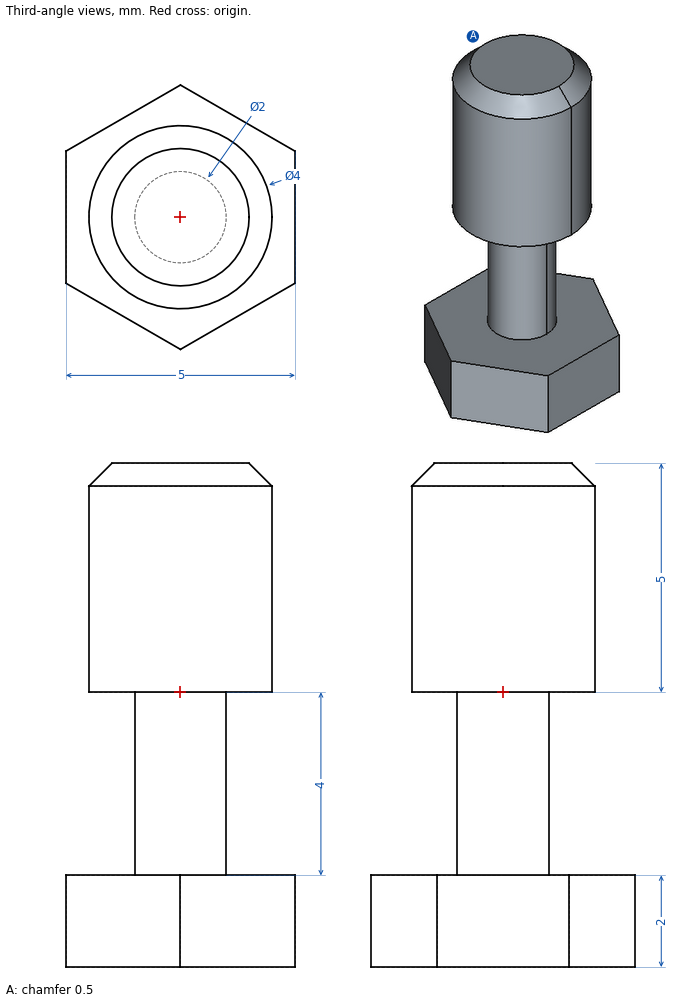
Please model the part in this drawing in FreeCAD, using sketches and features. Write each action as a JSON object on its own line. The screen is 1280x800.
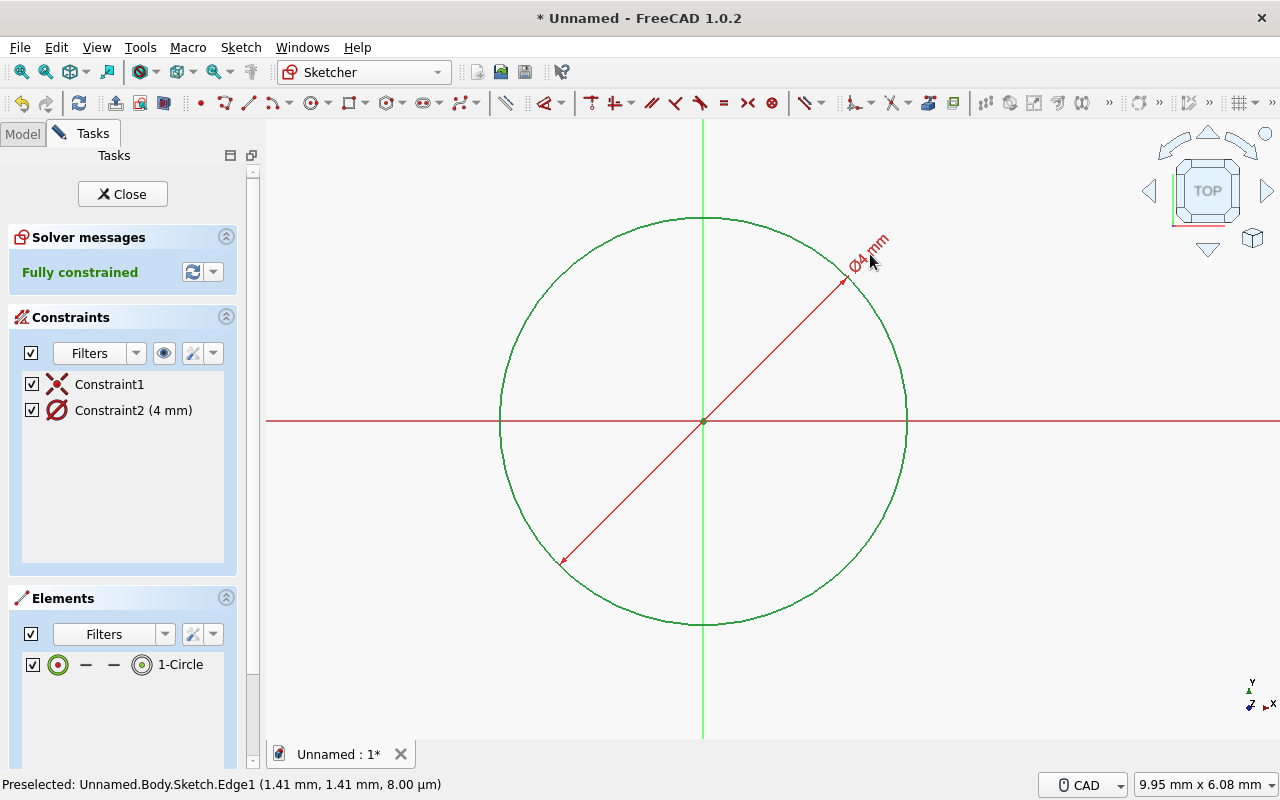
{"action": "left_click", "coordinate": [123, 194]}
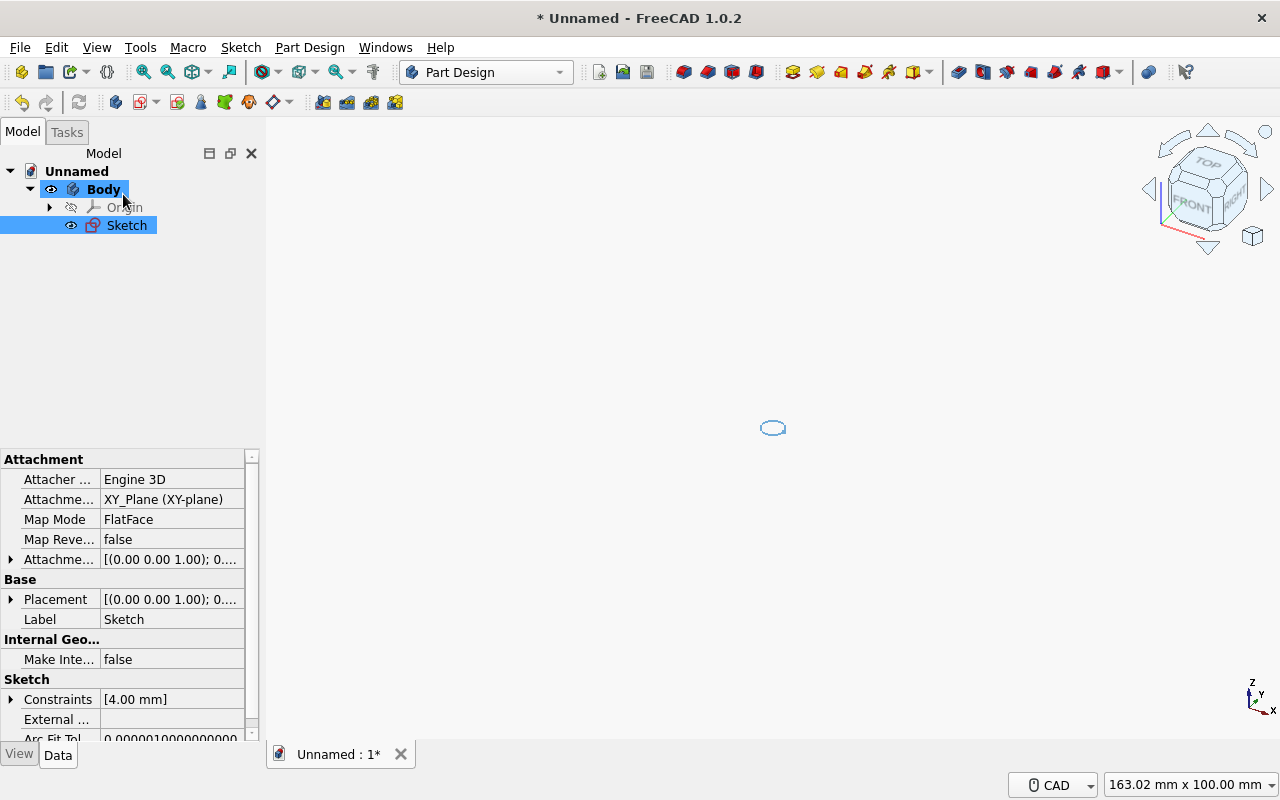
{"action": "left_click", "coordinate": [794, 72]}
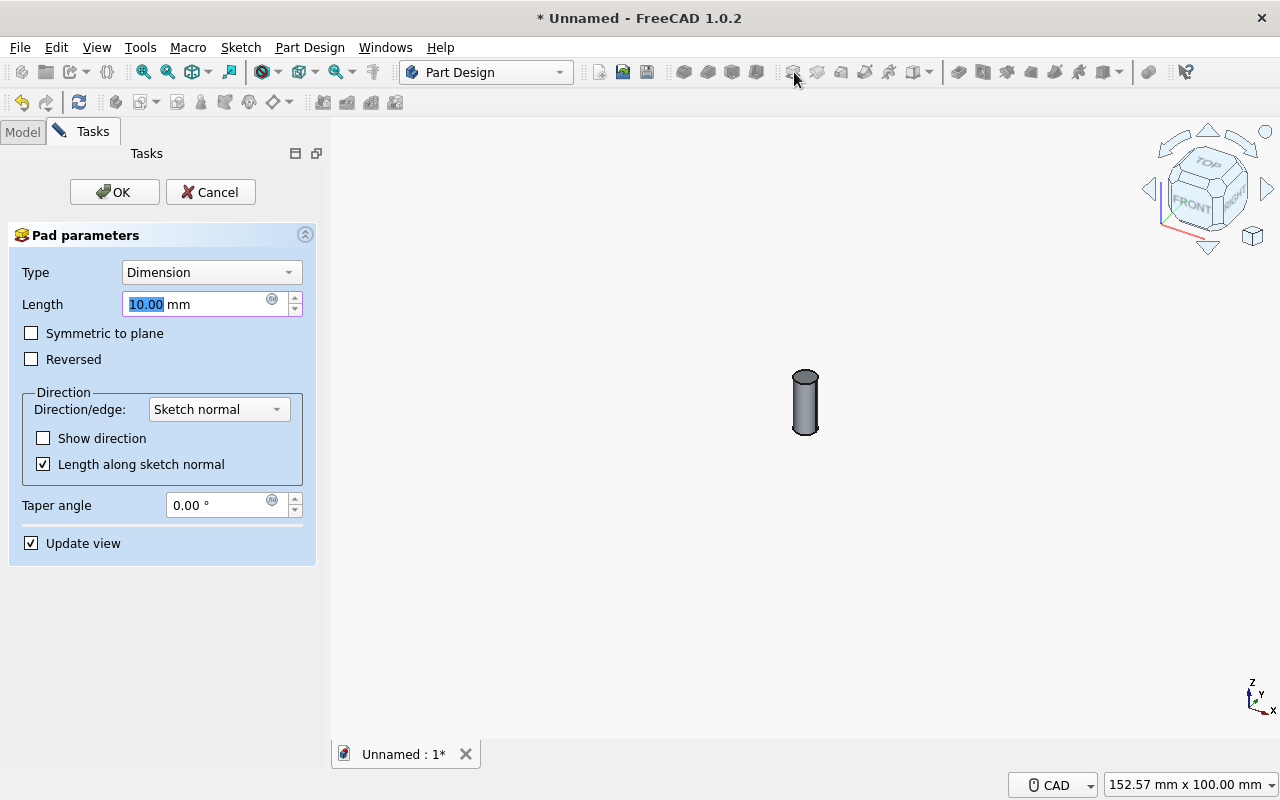
{"action": "type", "text": "5"}
{"action": "key", "text": "Tab"}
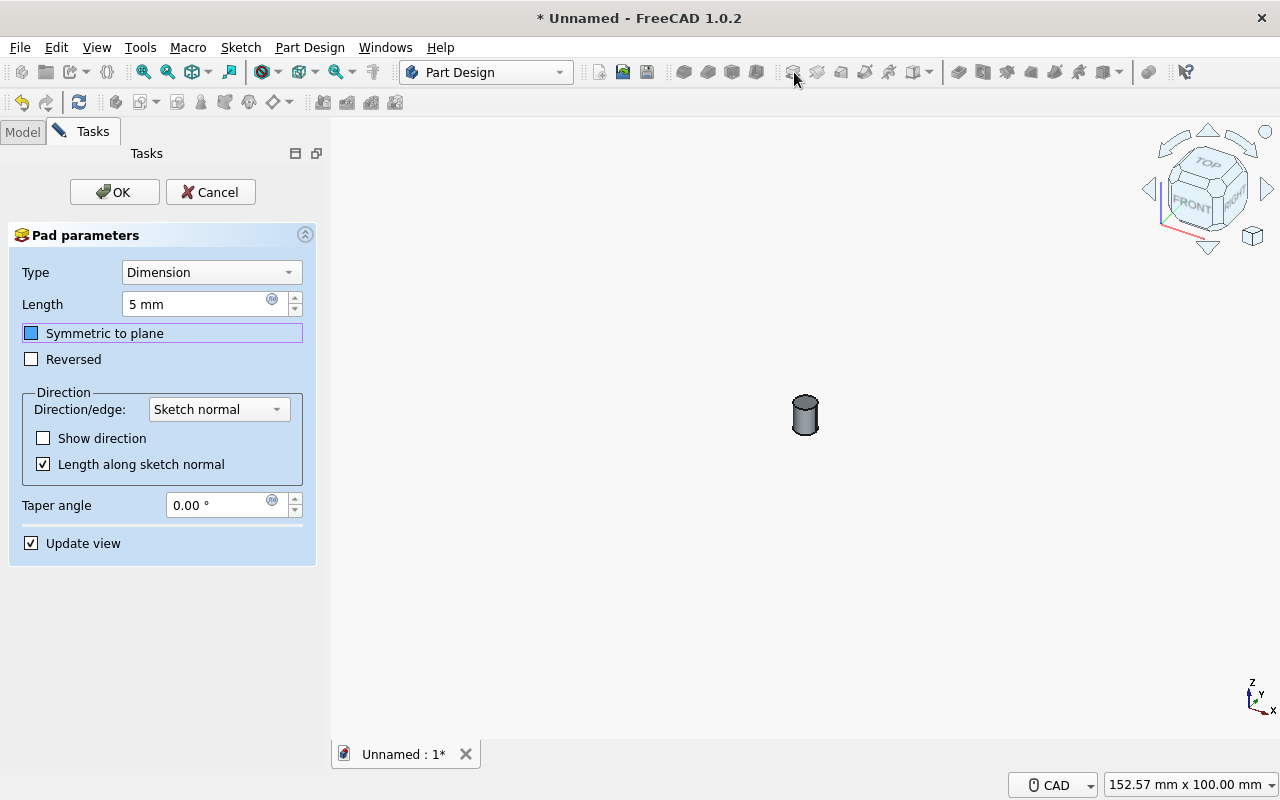
{"action": "left_click", "coordinate": [115, 192]}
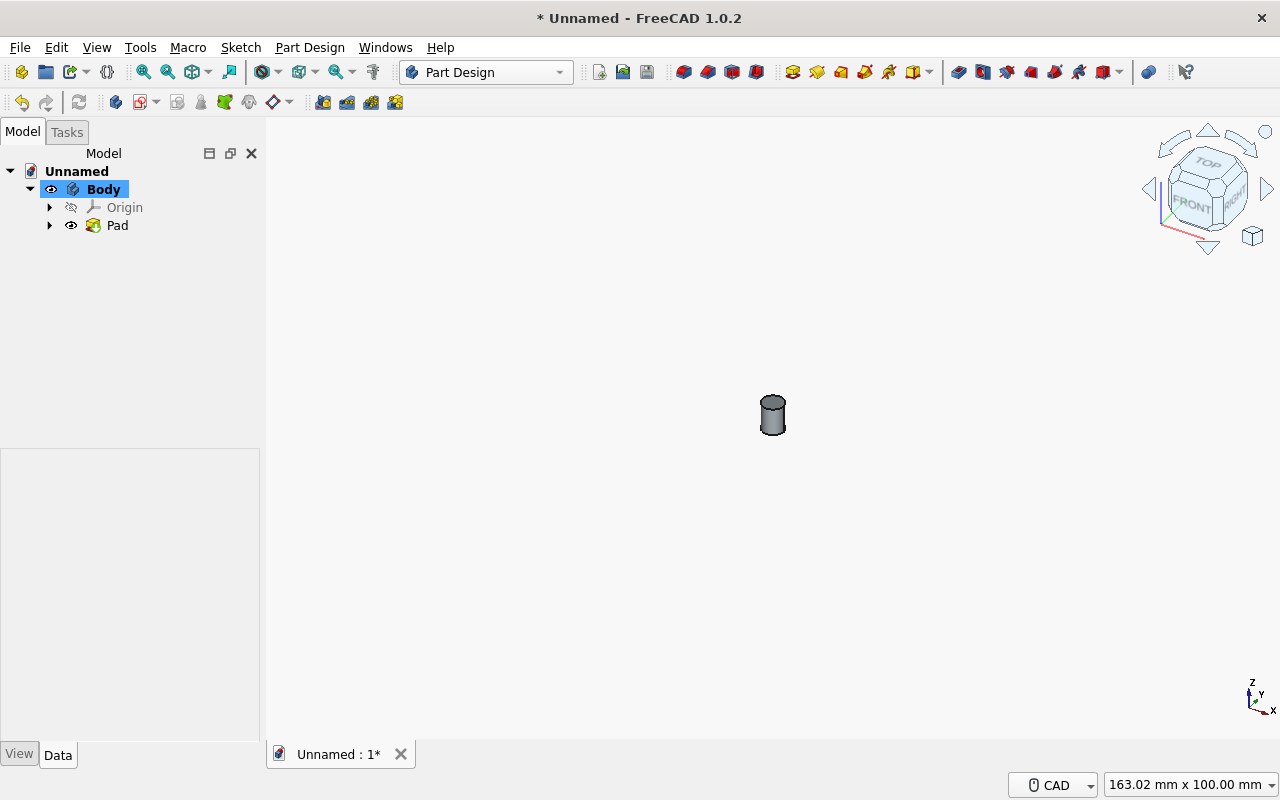
{"action": "left_click", "coordinate": [144, 72]}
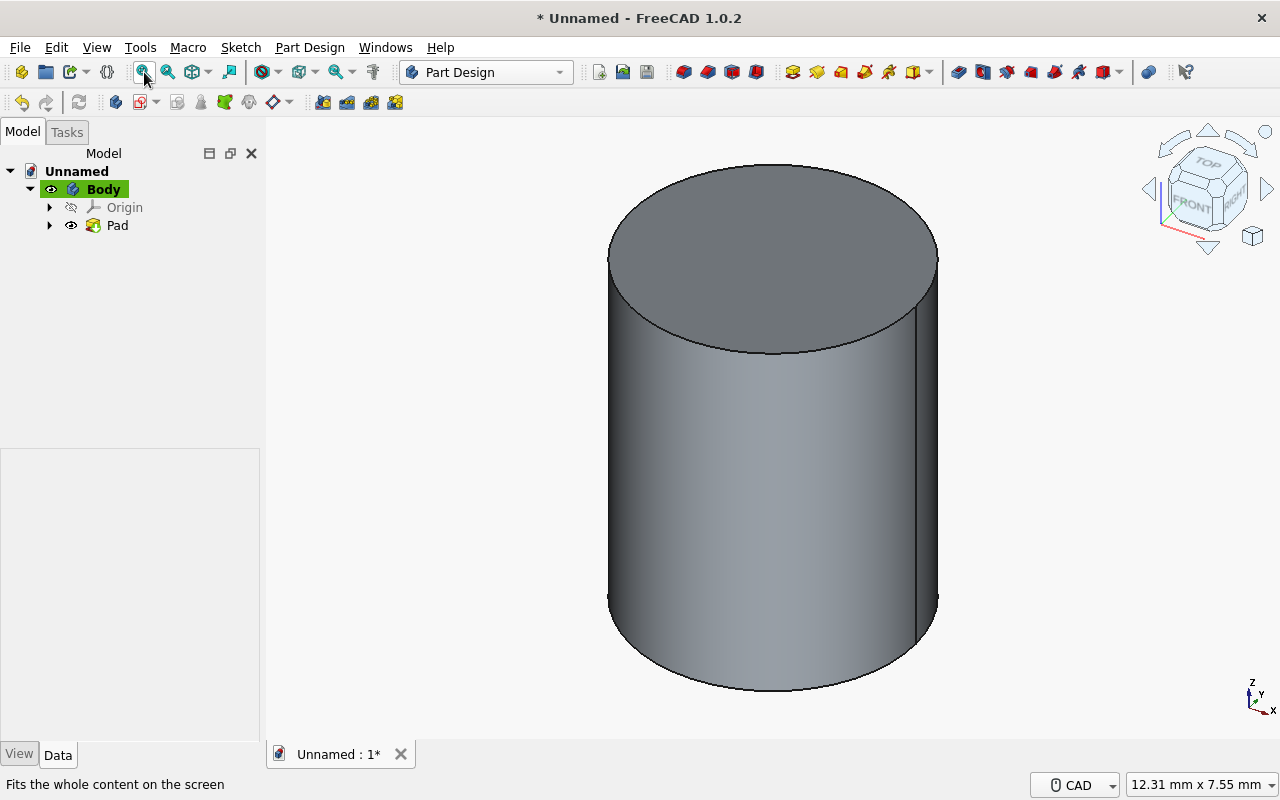
{"action": "left_click", "coordinate": [140, 102]}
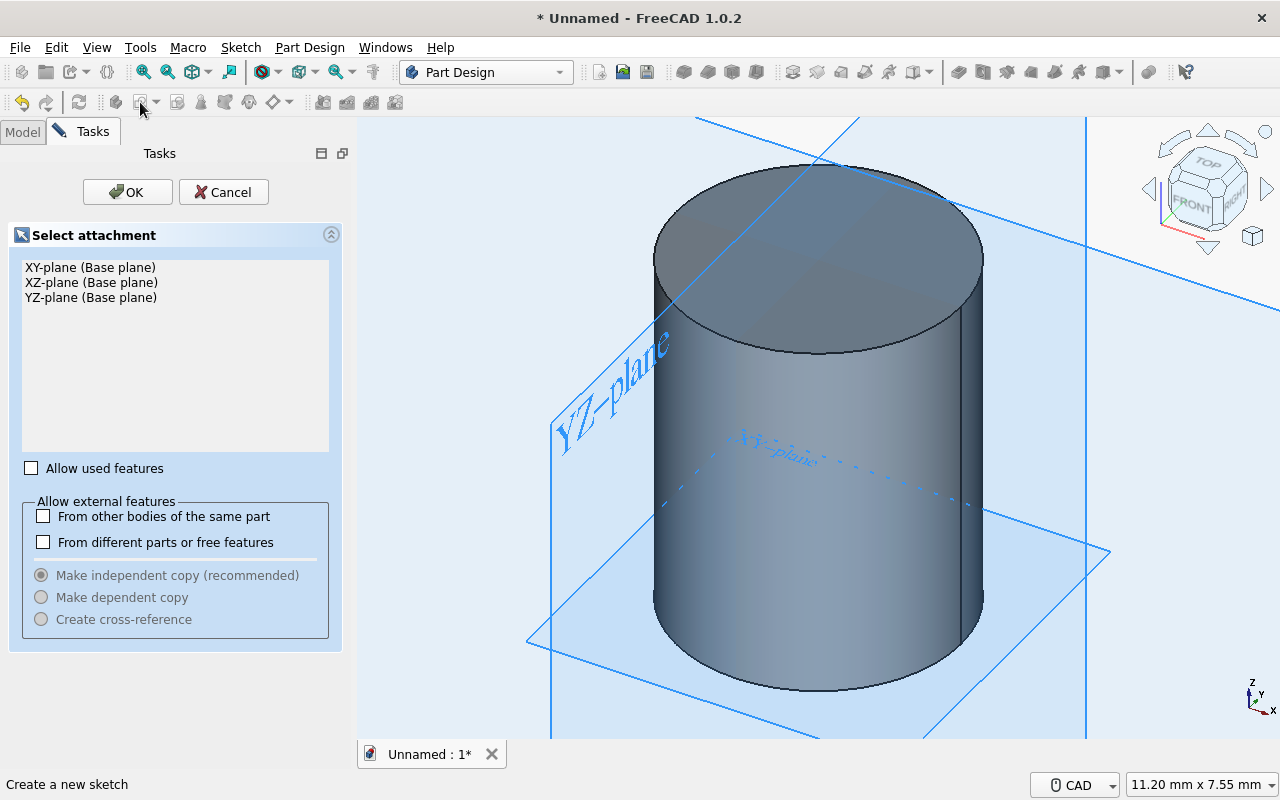
{"action": "left_click", "coordinate": [82, 268]}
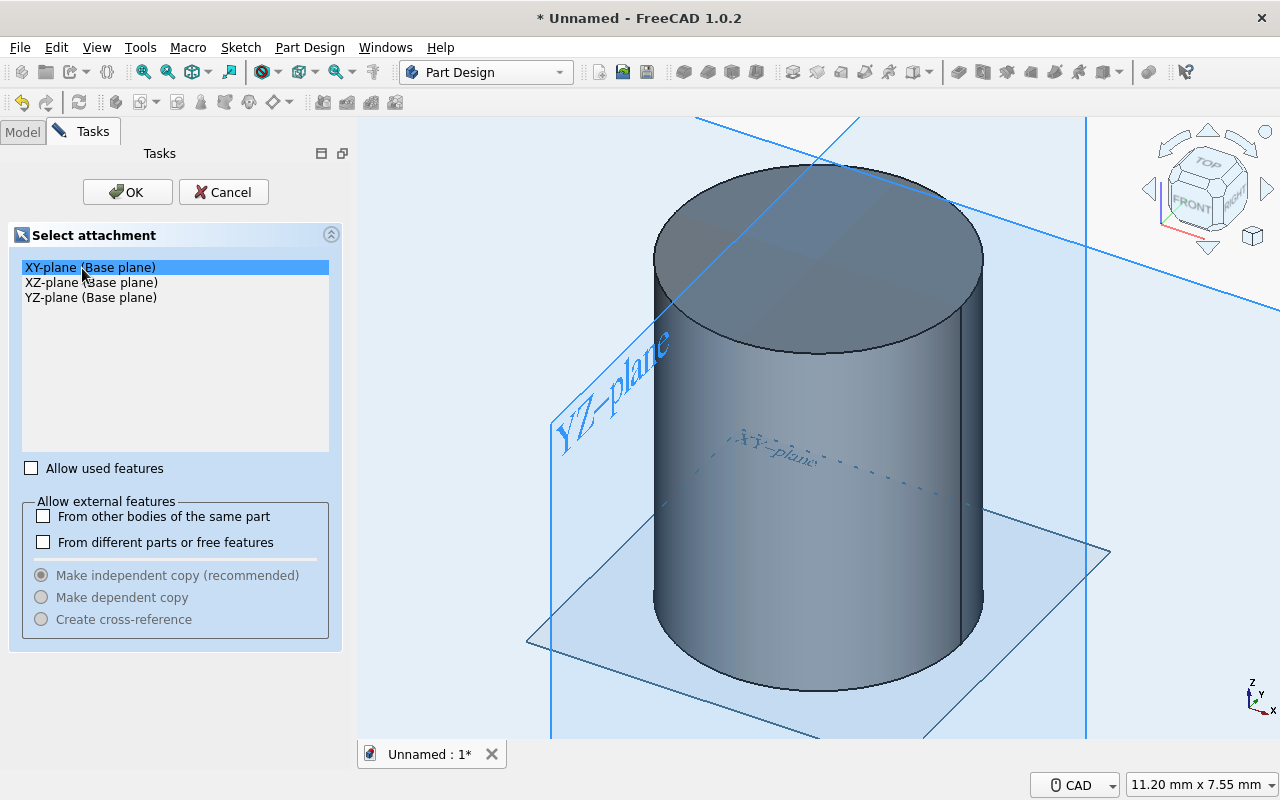
{"action": "left_click", "coordinate": [128, 192]}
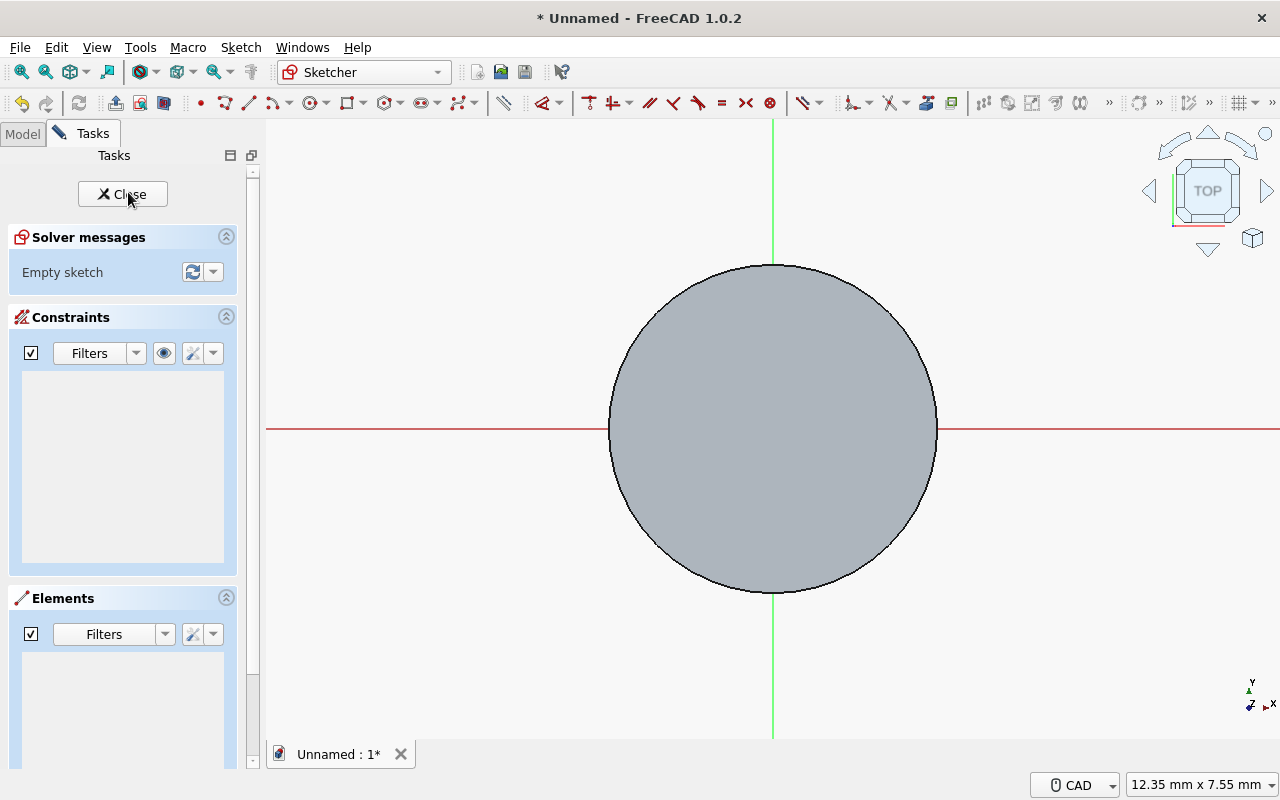
{"action": "left_click", "coordinate": [164, 104]}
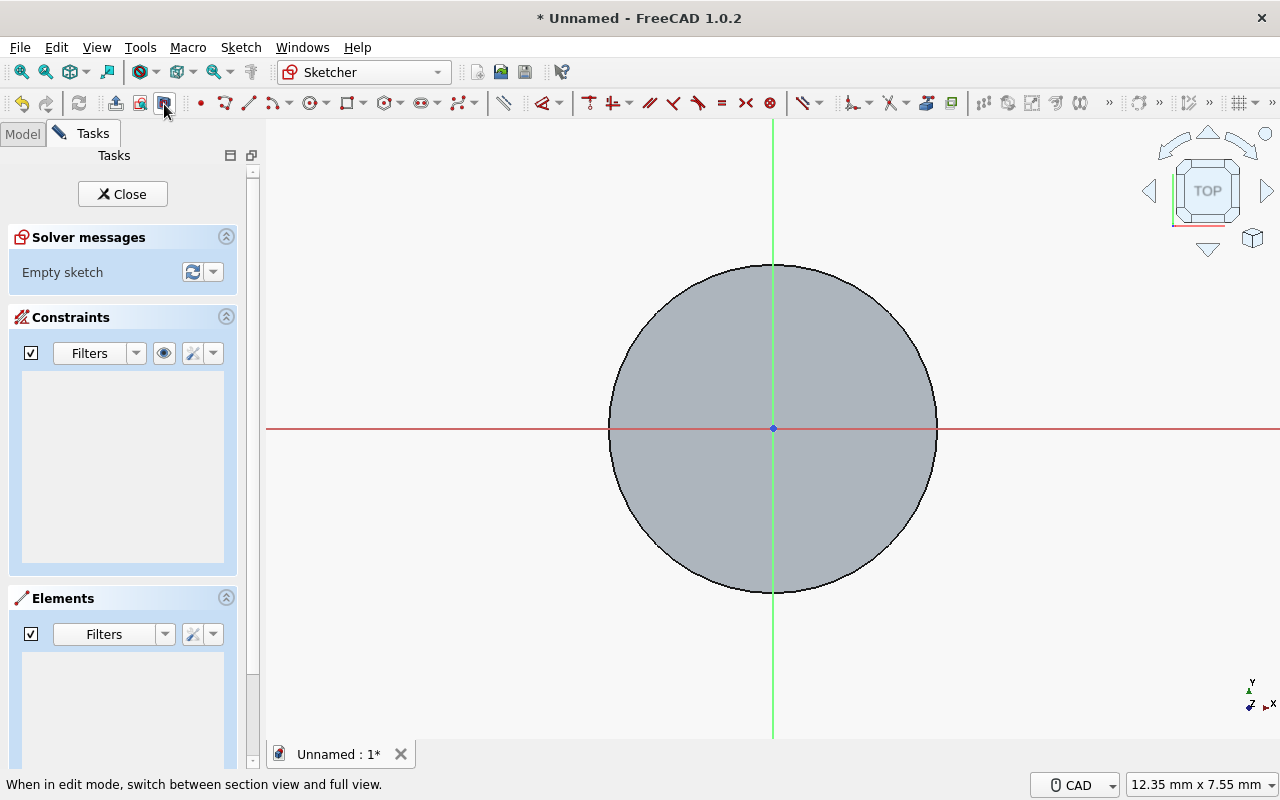
{"action": "scroll", "coordinate": [829, 429], "scroll_direction": "up", "scroll_amount": 4}